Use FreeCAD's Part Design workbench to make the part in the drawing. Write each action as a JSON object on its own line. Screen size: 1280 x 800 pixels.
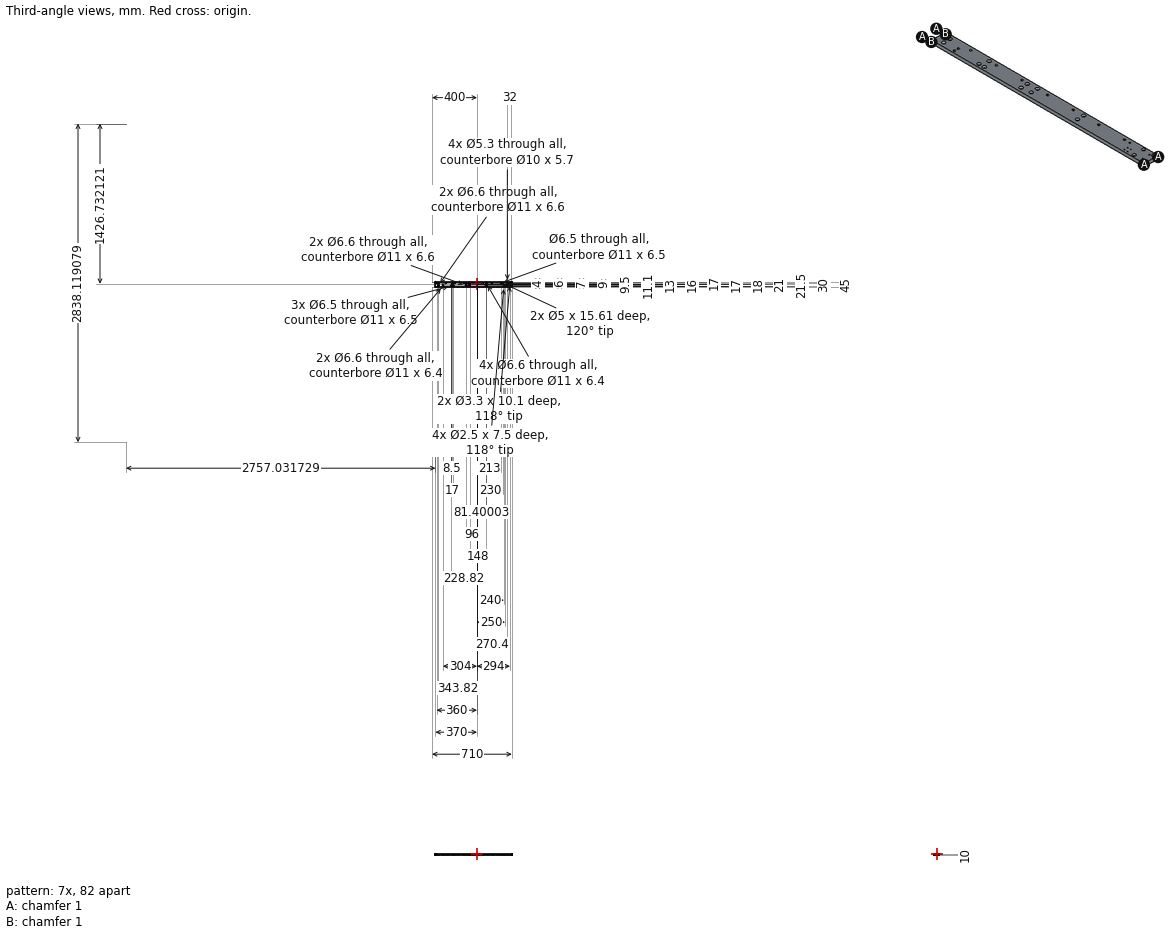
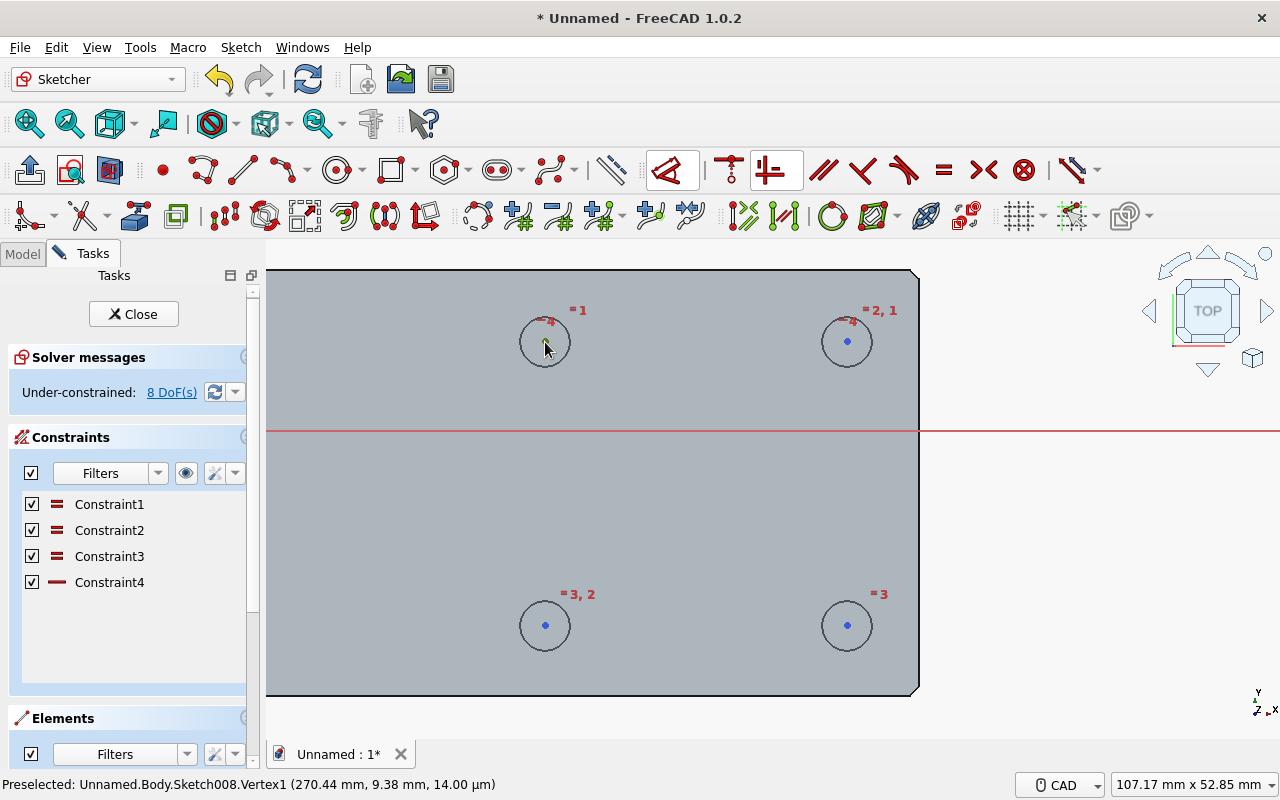
{"action": "left_click", "coordinate": [545, 626]}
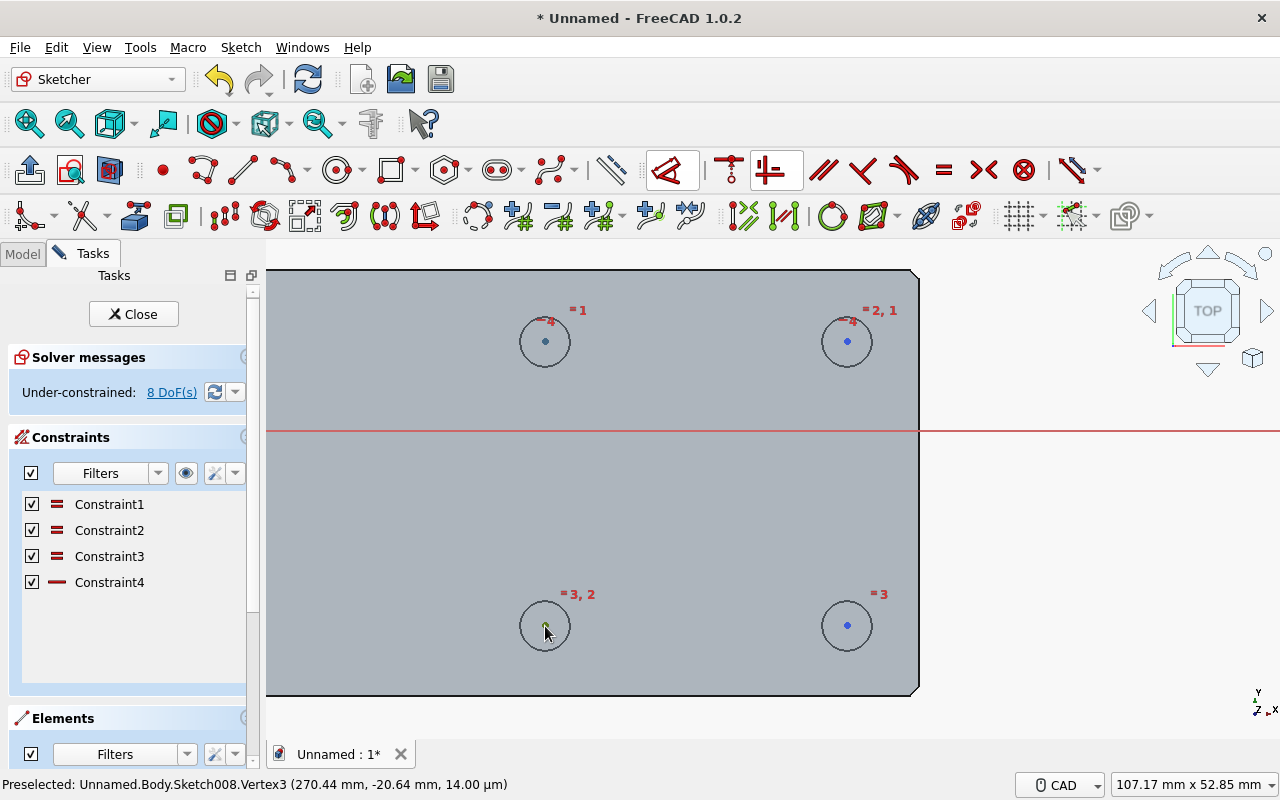
{"action": "key", "text": "v"}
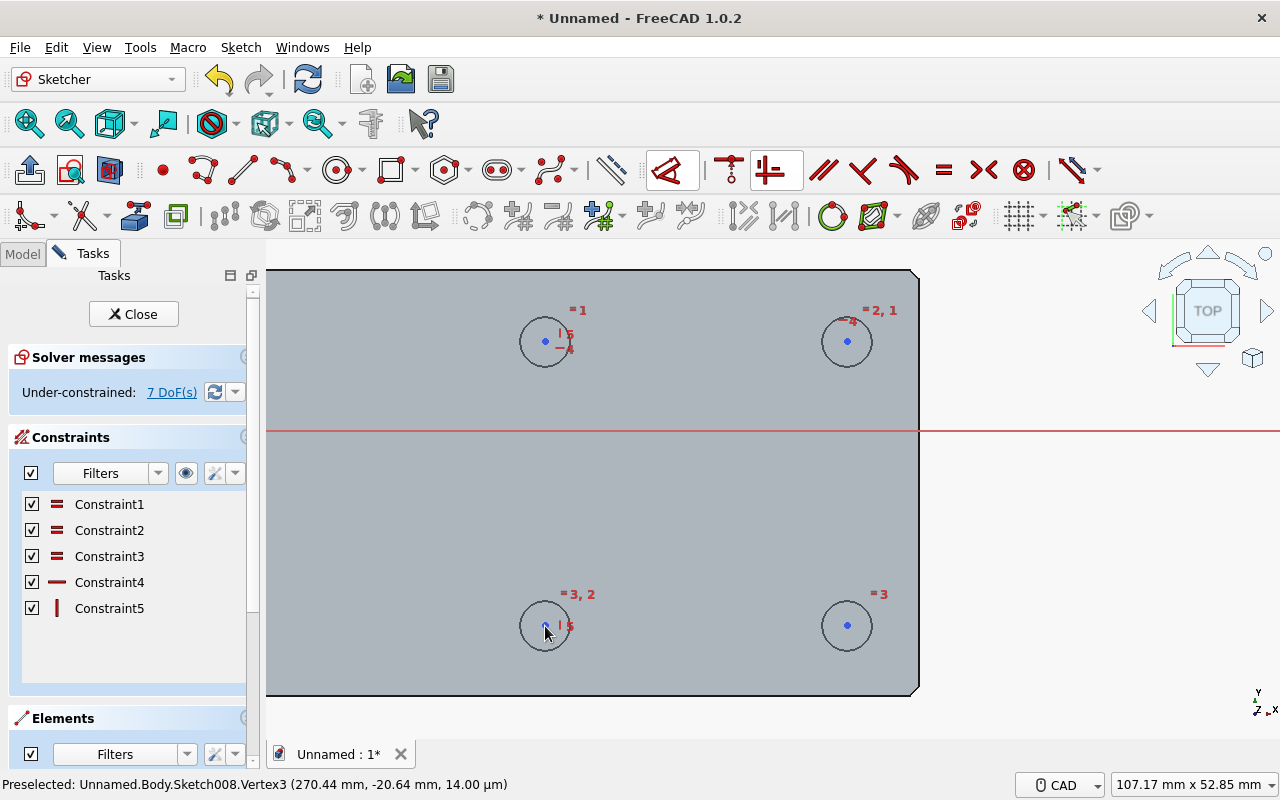
{"action": "left_click", "coordinate": [847, 342]}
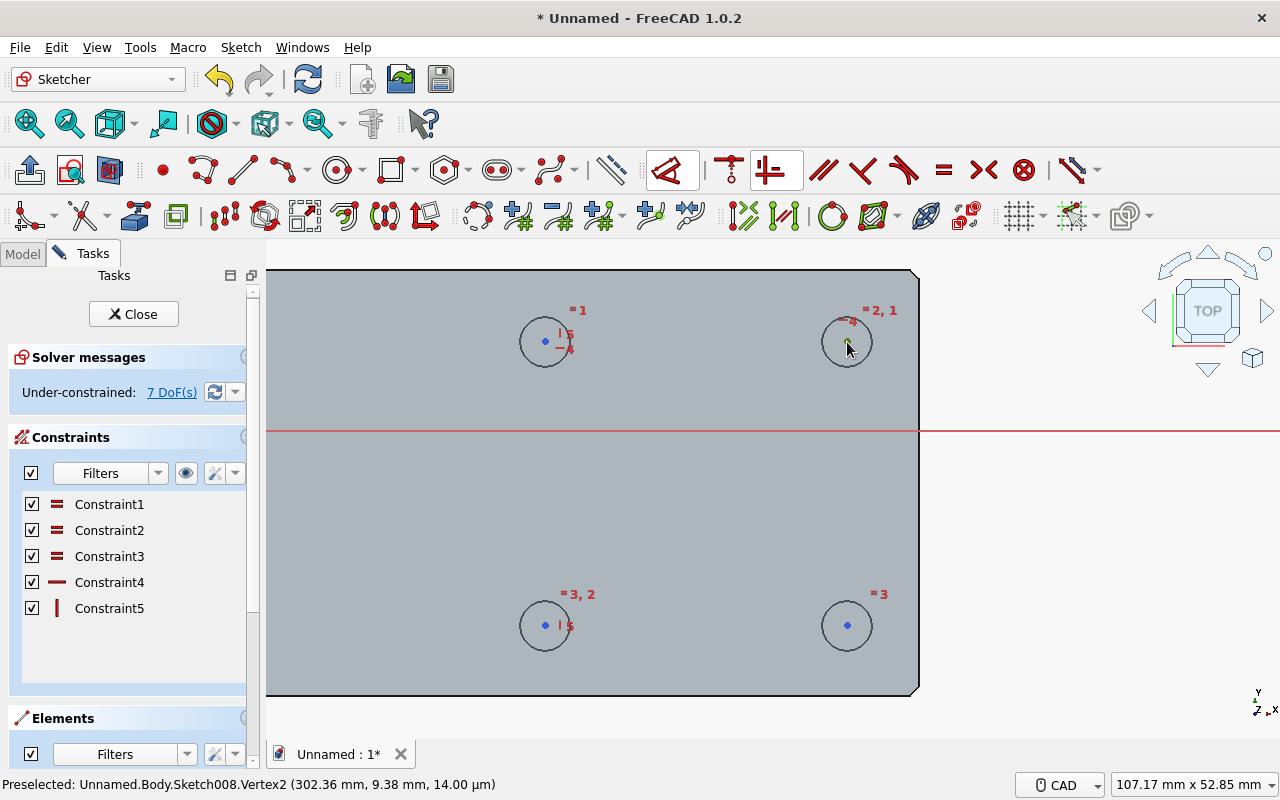
{"action": "left_click", "coordinate": [847, 626]}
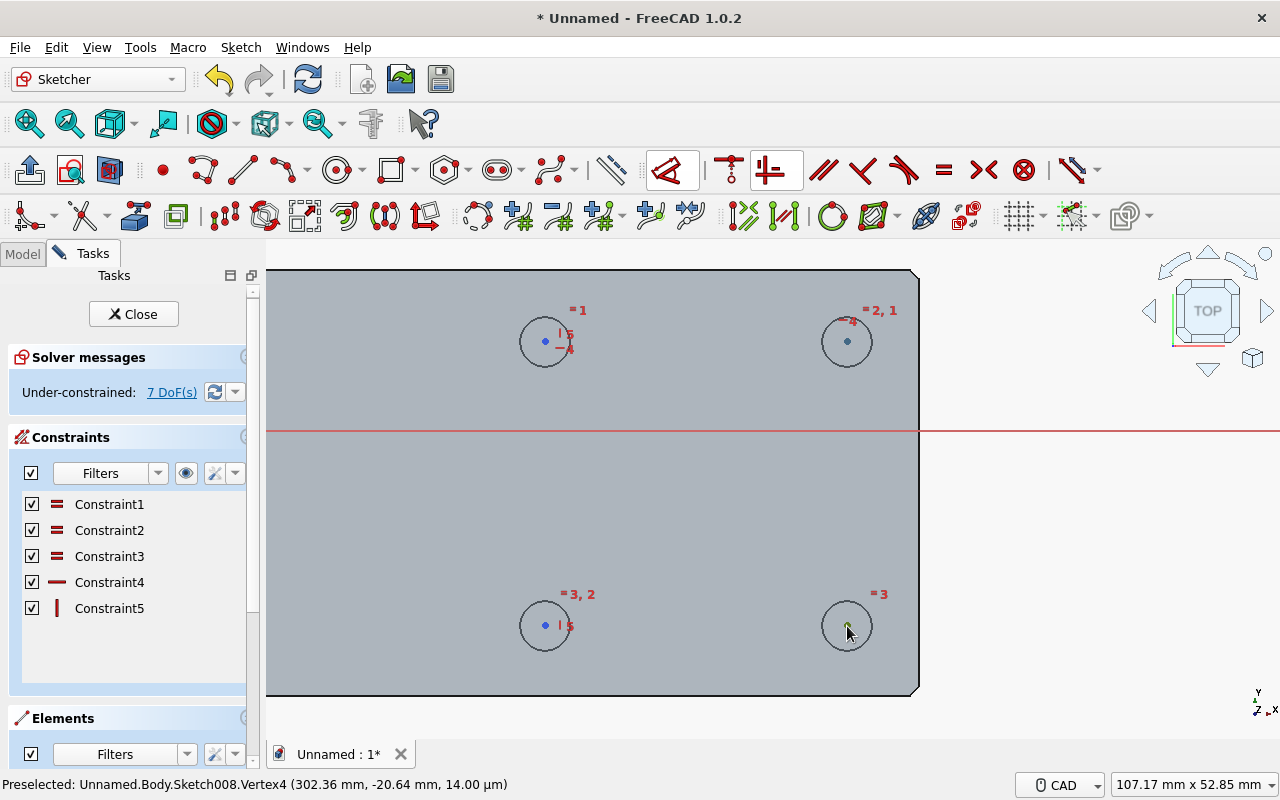
{"action": "left_click", "coordinate": [798, 170]}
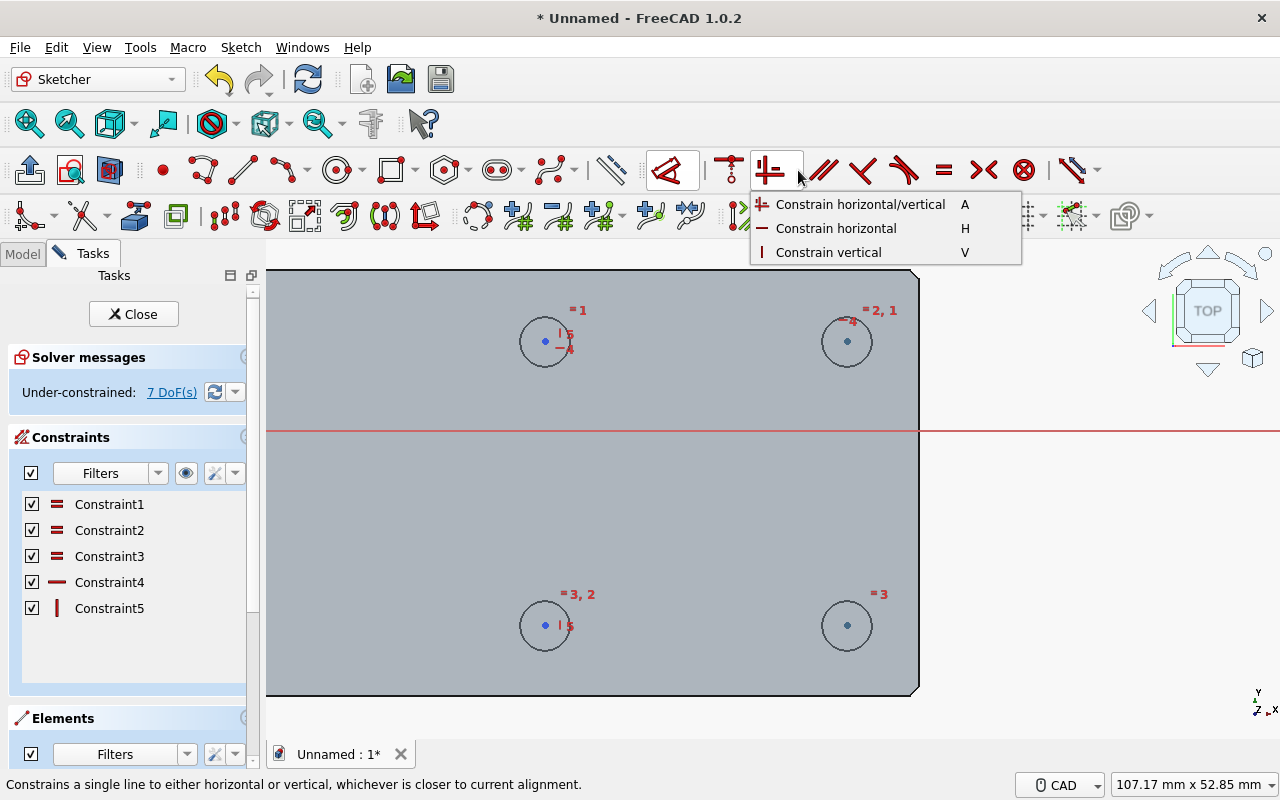
{"action": "left_click", "coordinate": [886, 252]}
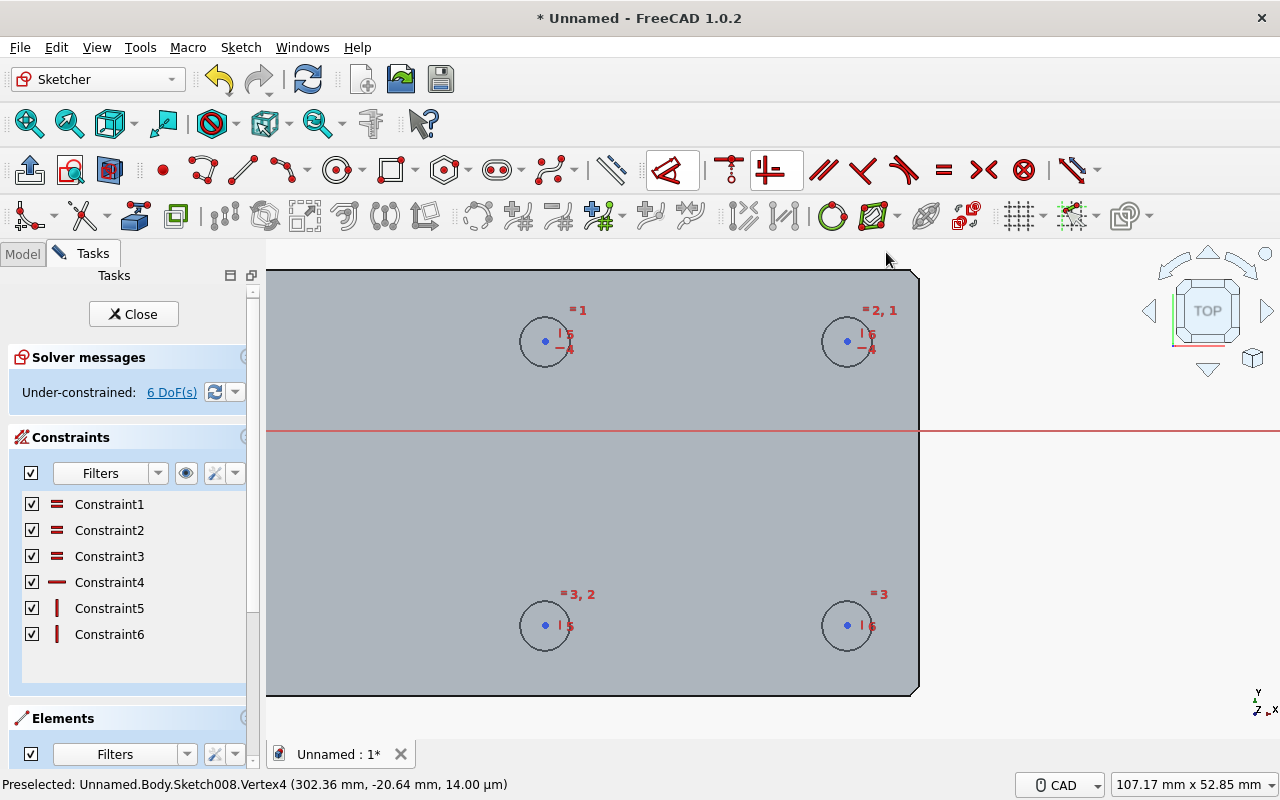
{"action": "left_click", "coordinate": [545, 626]}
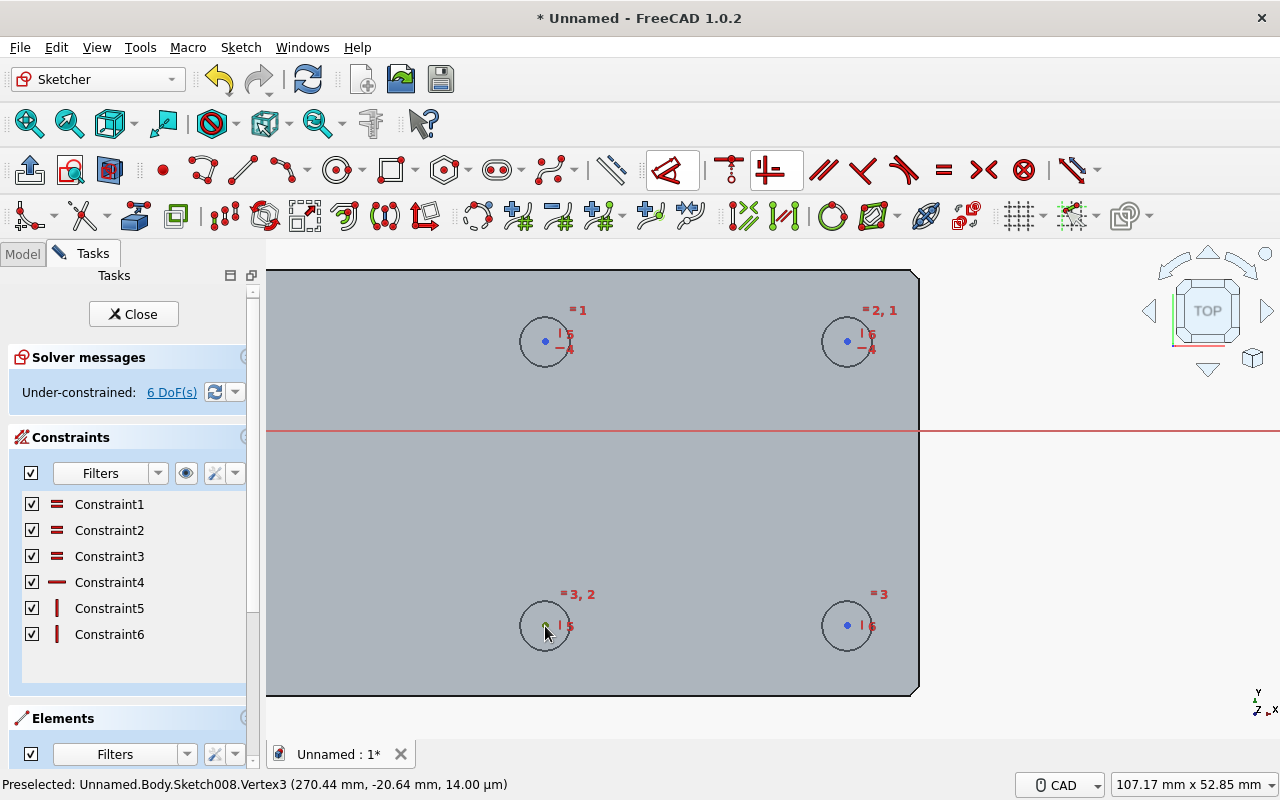
{"action": "left_click", "coordinate": [847, 626]}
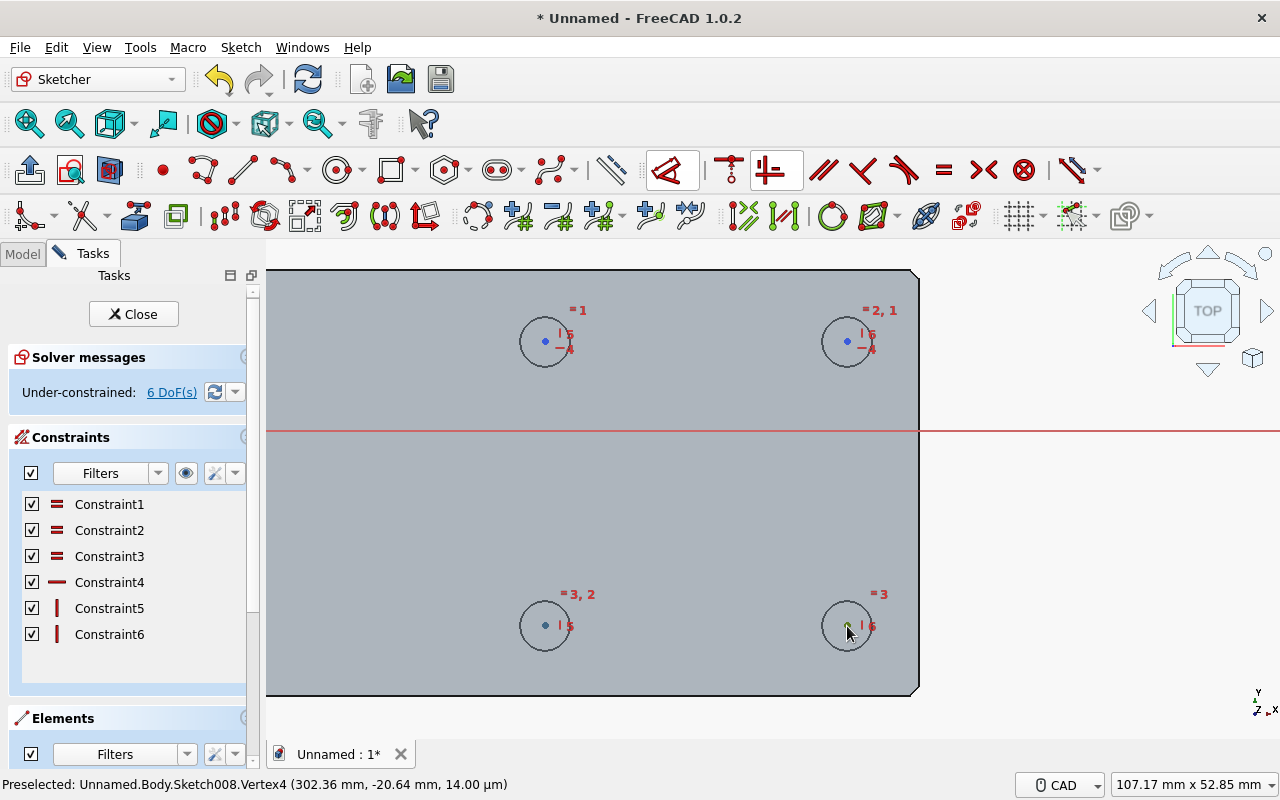
{"action": "left_click", "coordinate": [798, 170]}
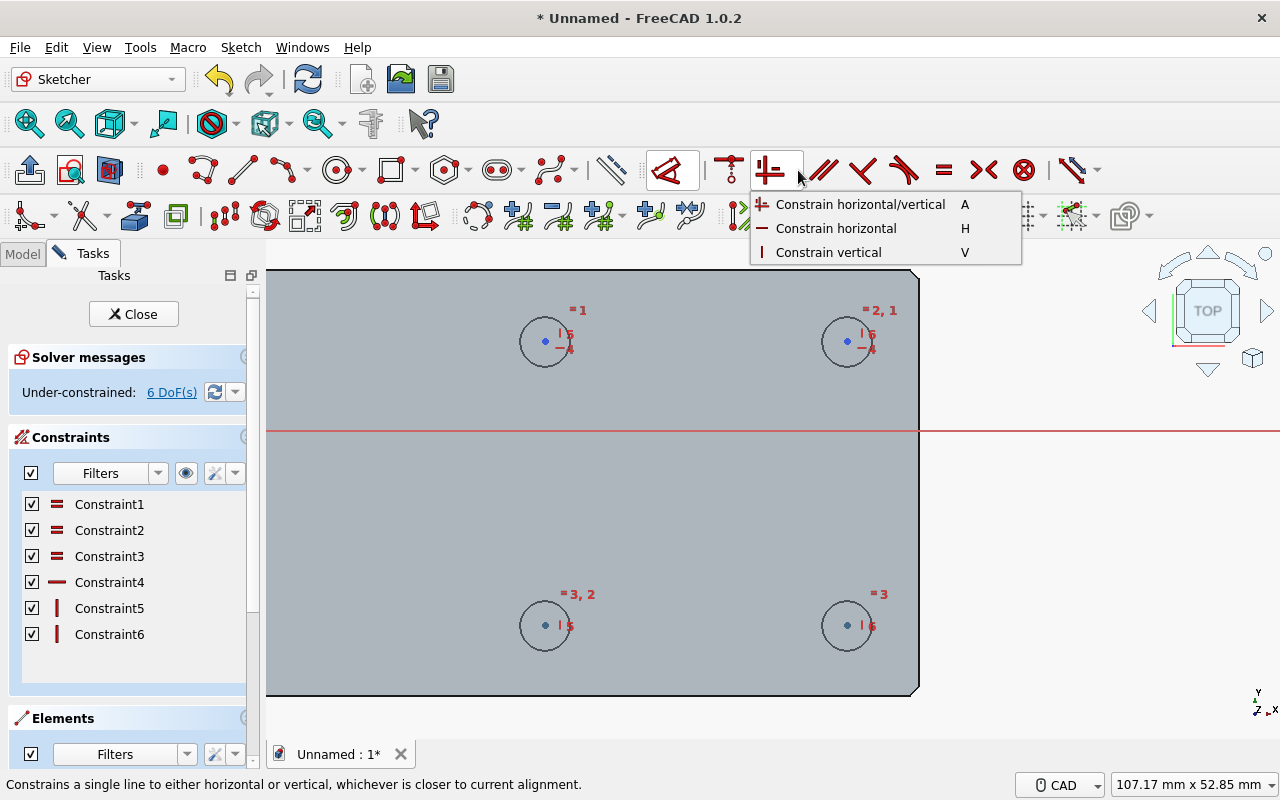
{"action": "left_click", "coordinate": [886, 228]}